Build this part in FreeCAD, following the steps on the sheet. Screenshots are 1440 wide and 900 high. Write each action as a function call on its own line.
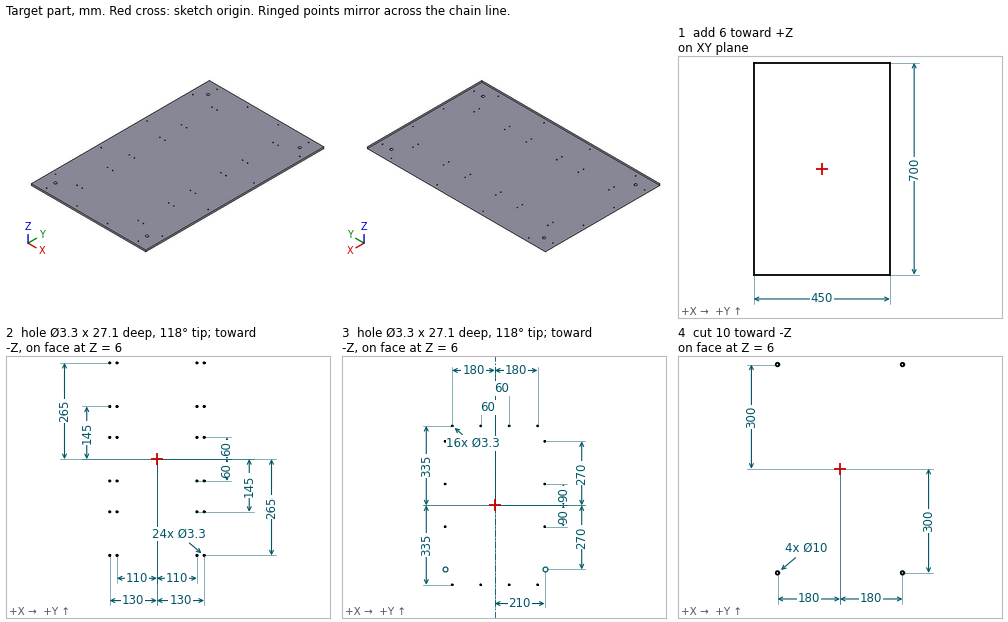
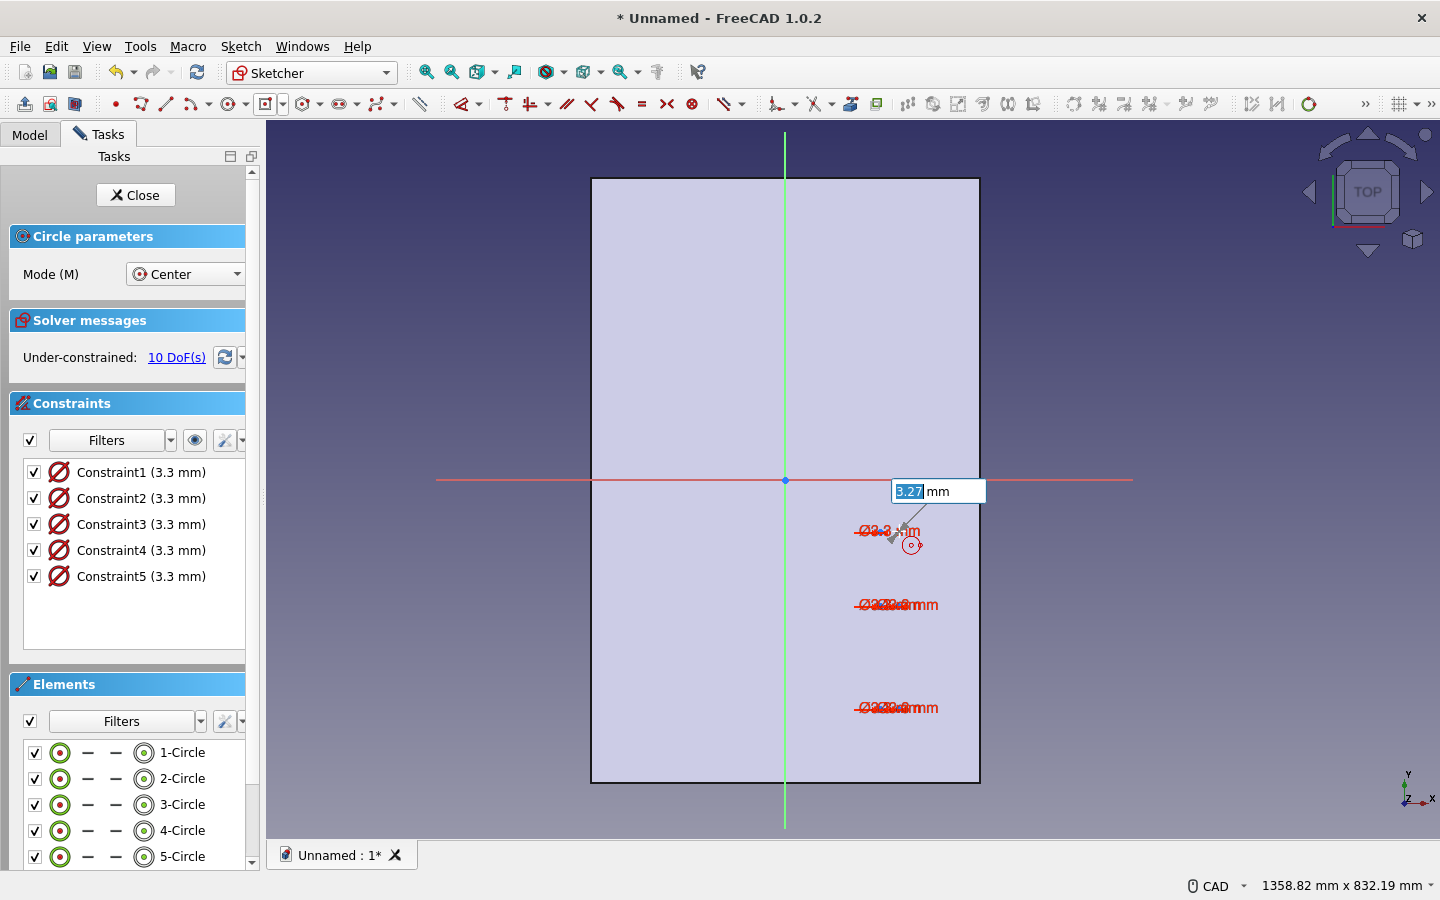
text(3.3)
key(Return)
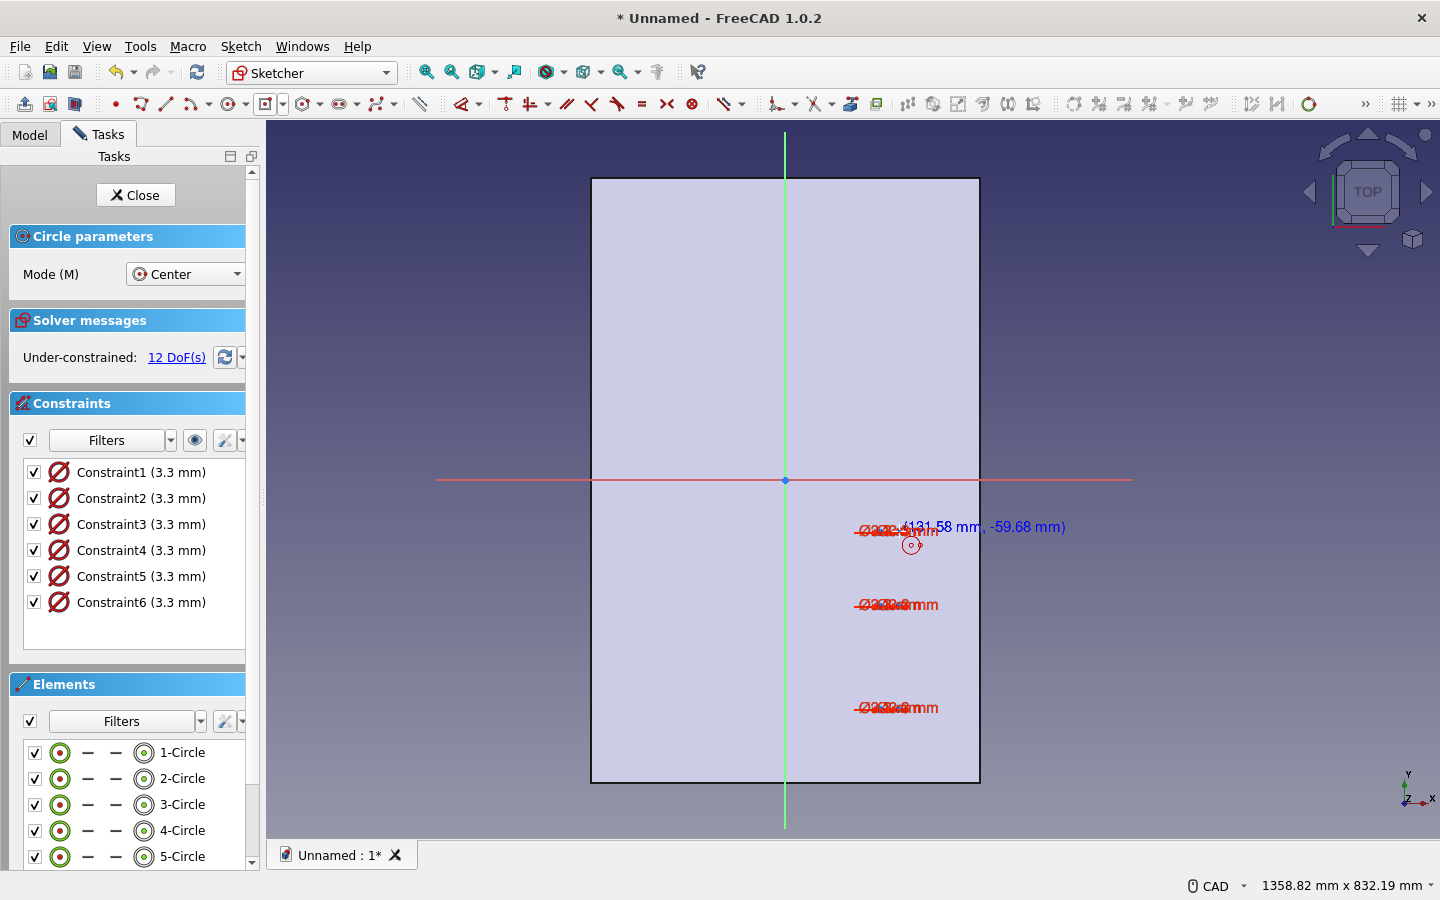
scroll(898, 429, up, 14)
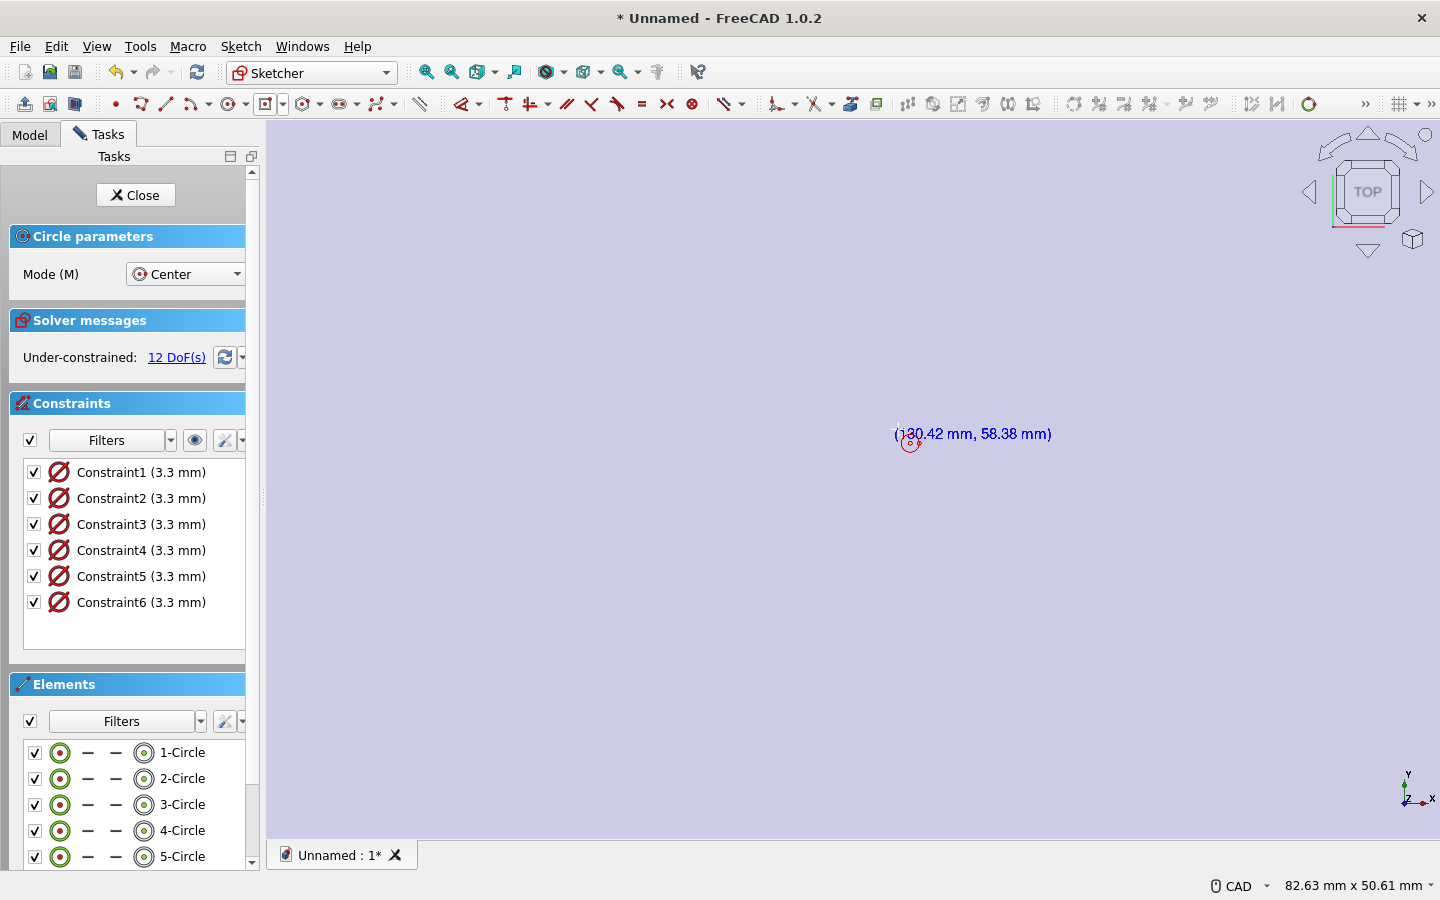
scroll(898, 428, down, 14)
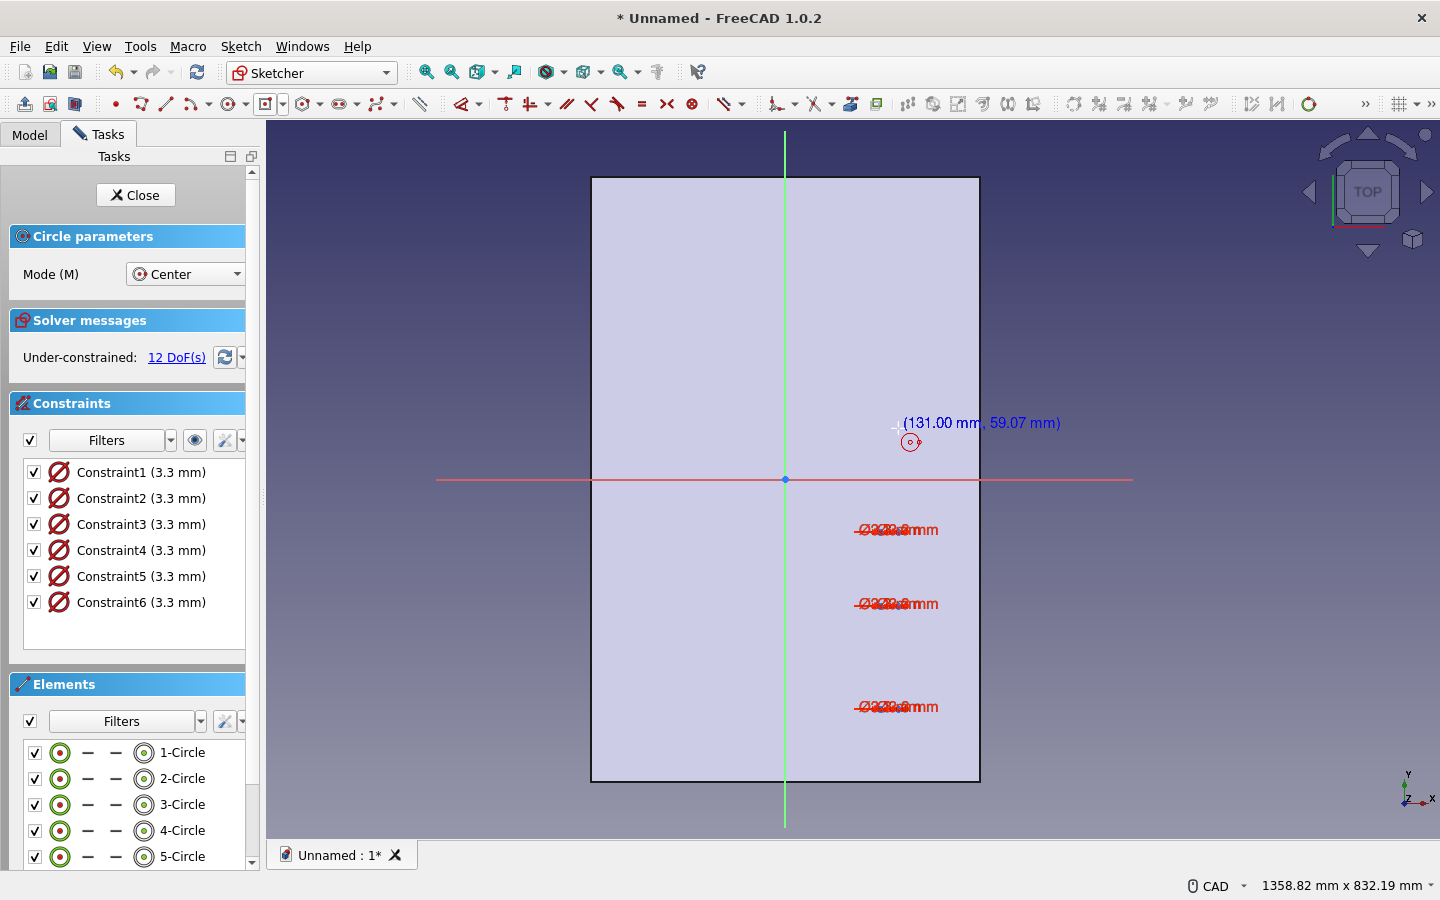
click(898, 428)
move(899, 427)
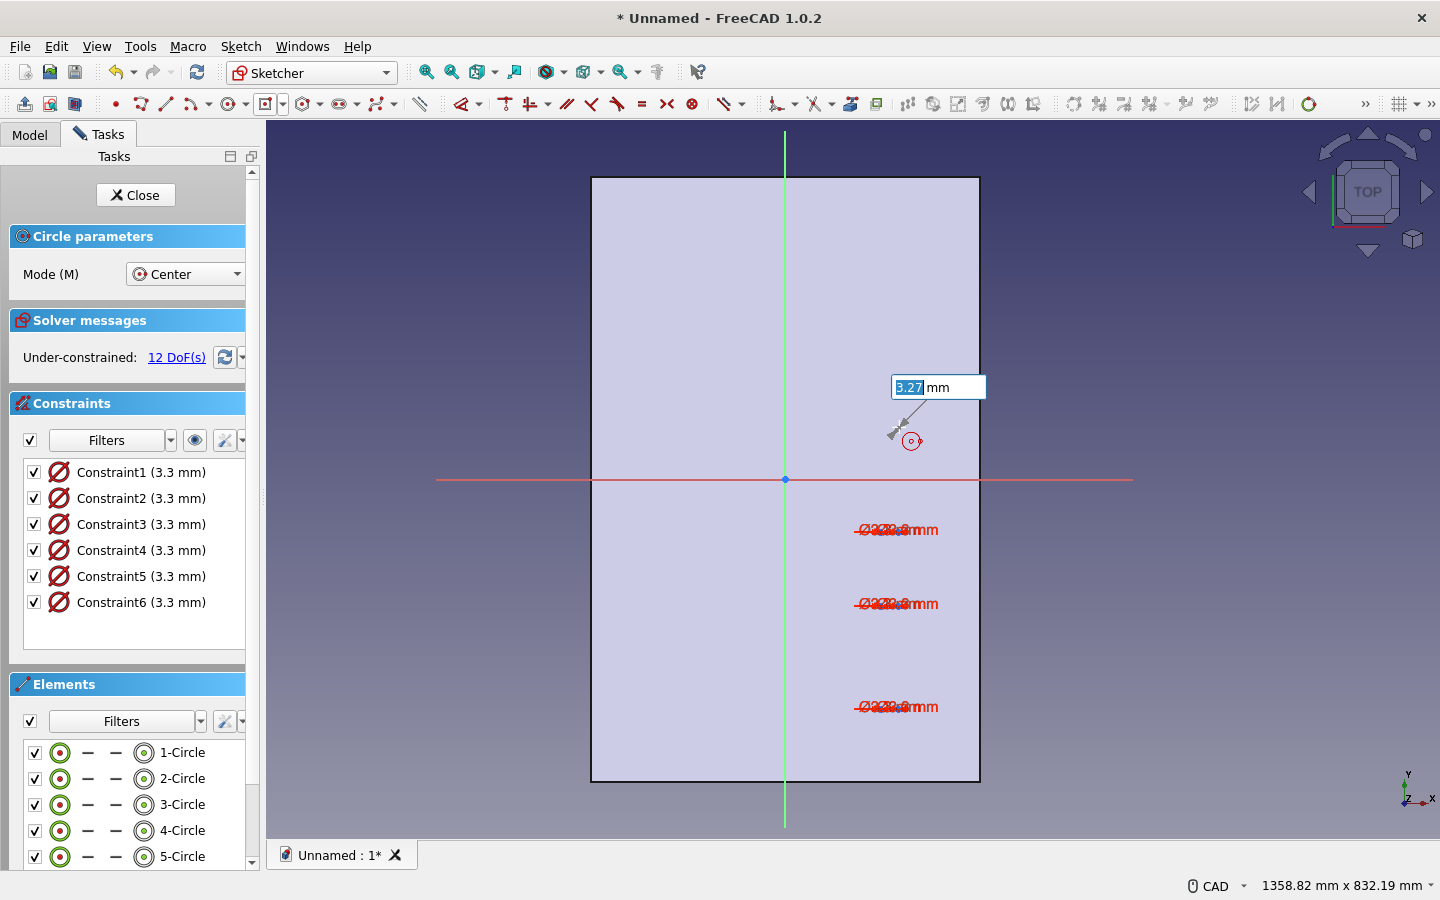
text(3.3)
key(Return)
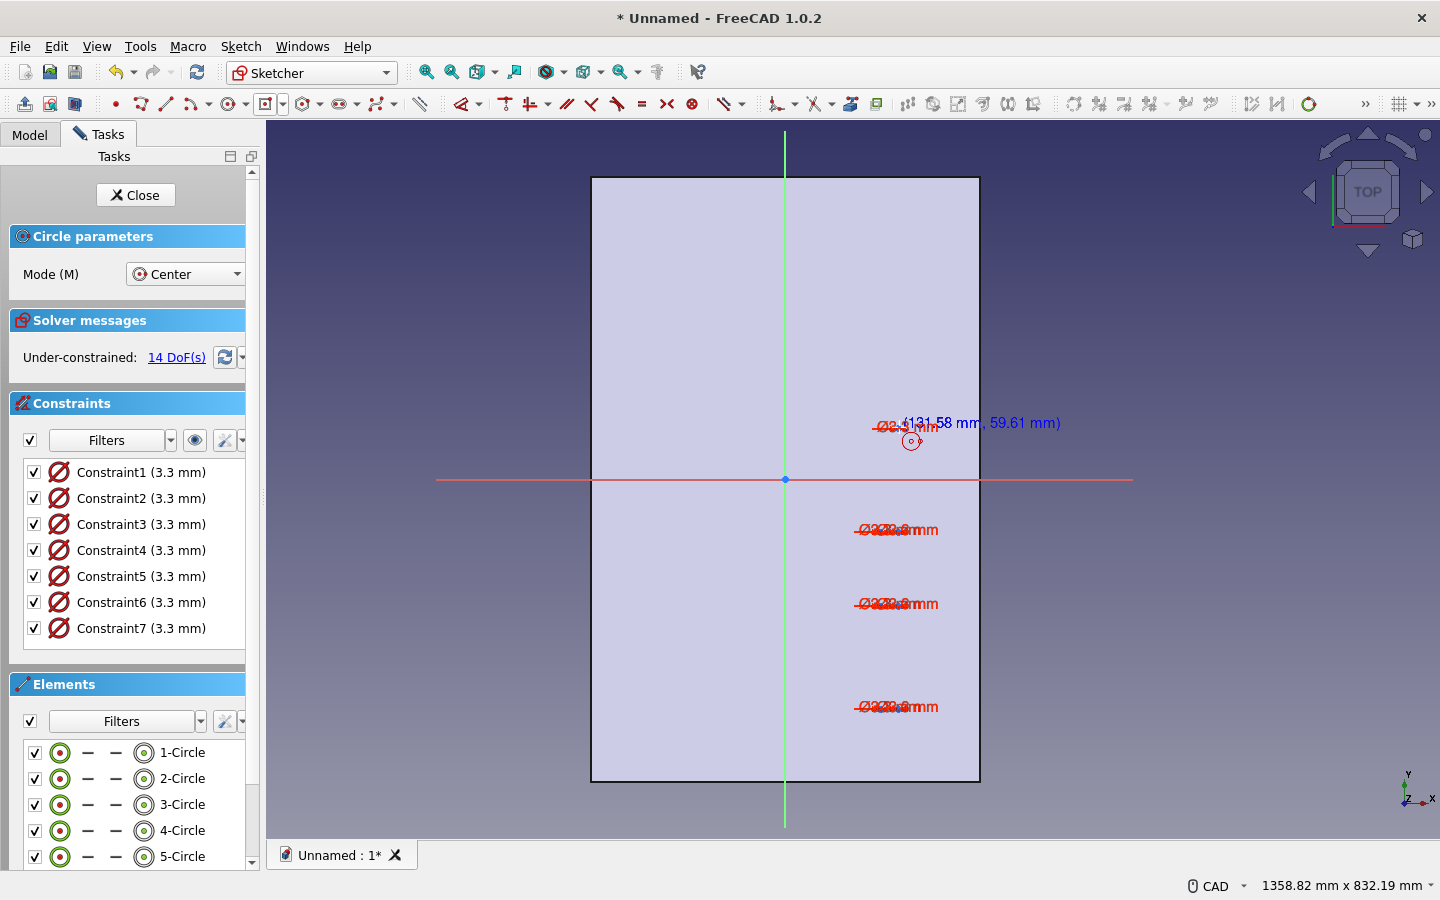
scroll(880, 428, up, 14)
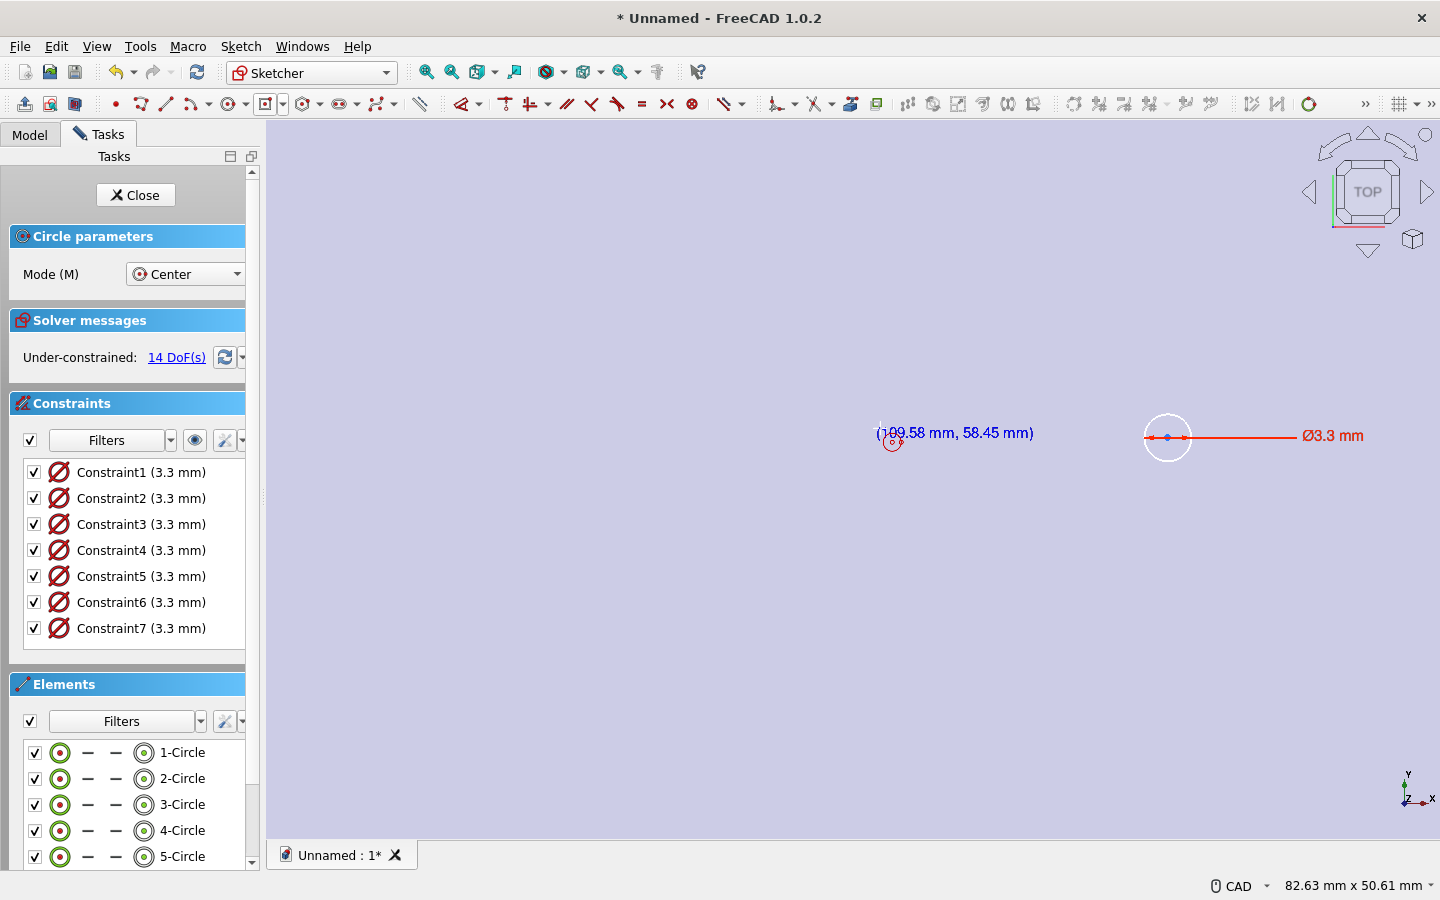
scroll(880, 428, down, 14)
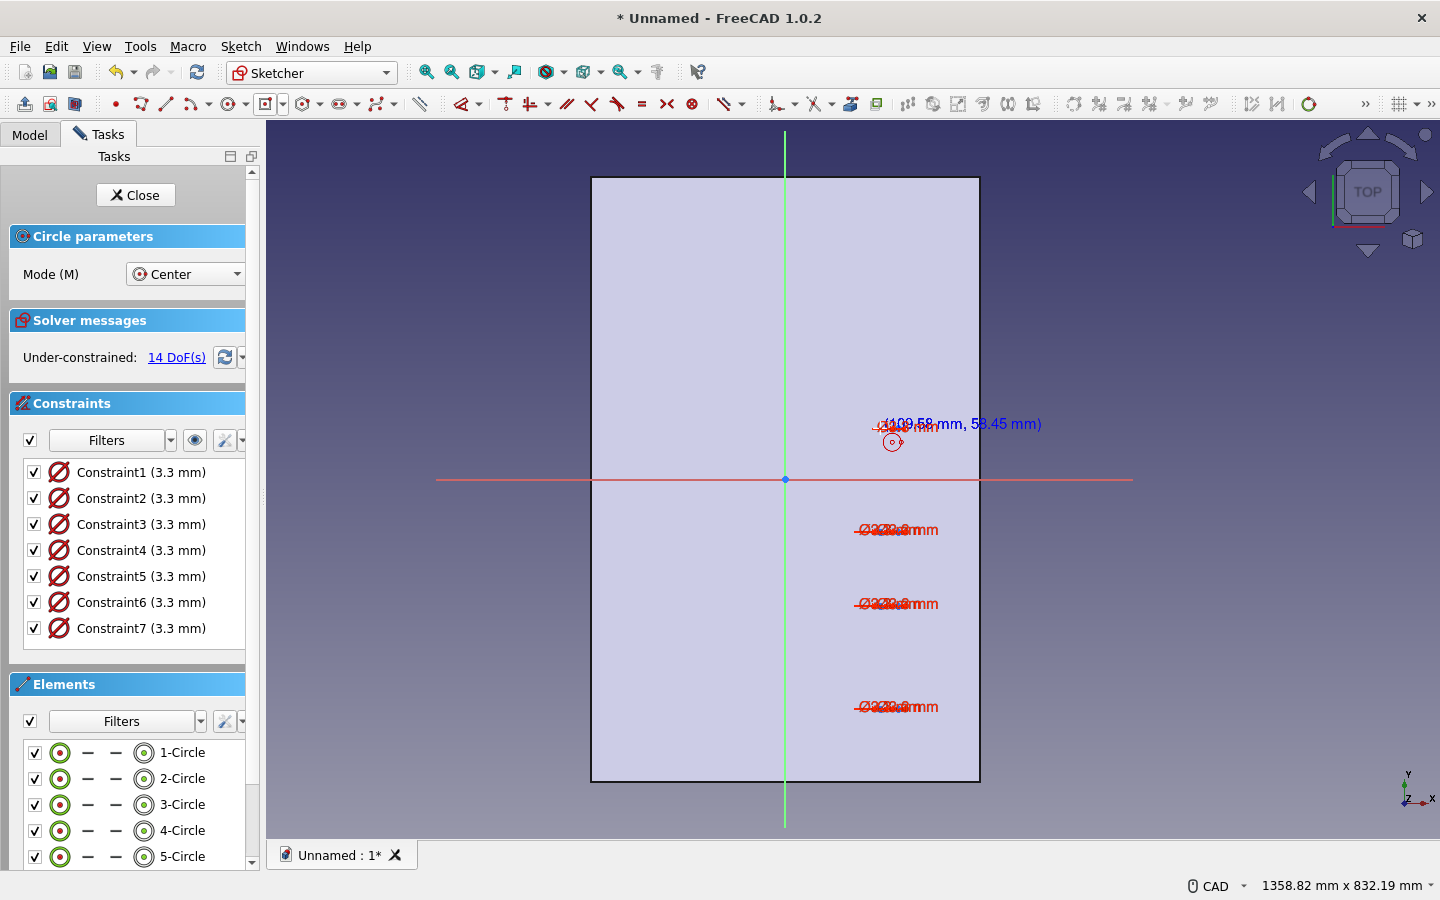
click(880, 428)
move(881, 427)